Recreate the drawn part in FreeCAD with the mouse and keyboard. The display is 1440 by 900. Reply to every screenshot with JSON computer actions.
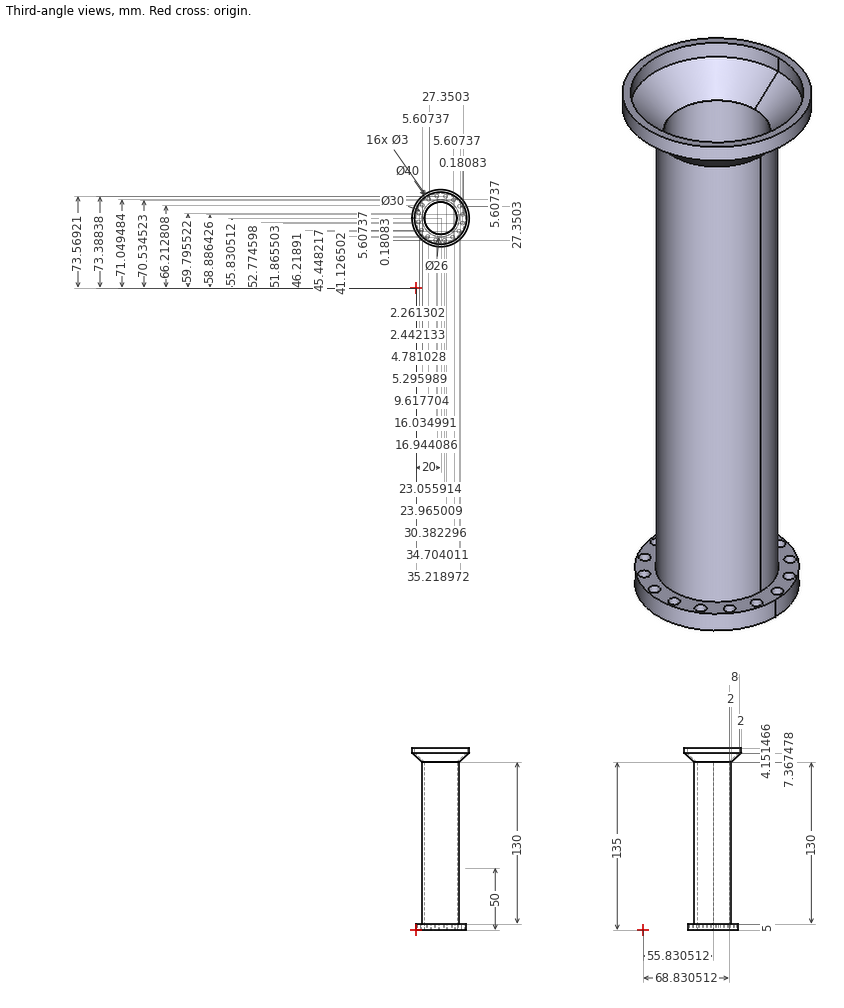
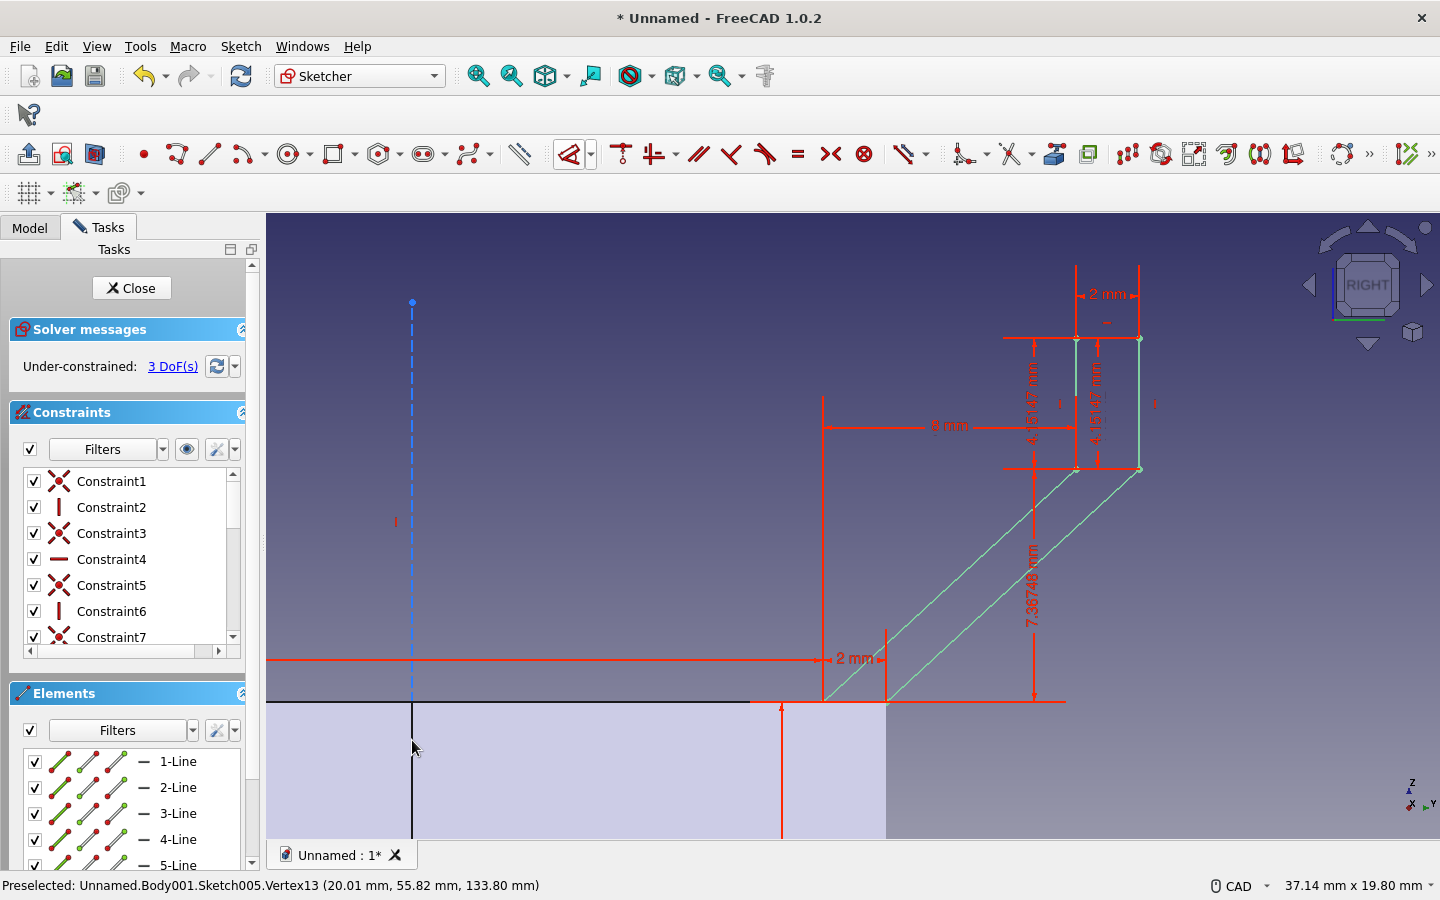
{"action": "key", "text": "l"}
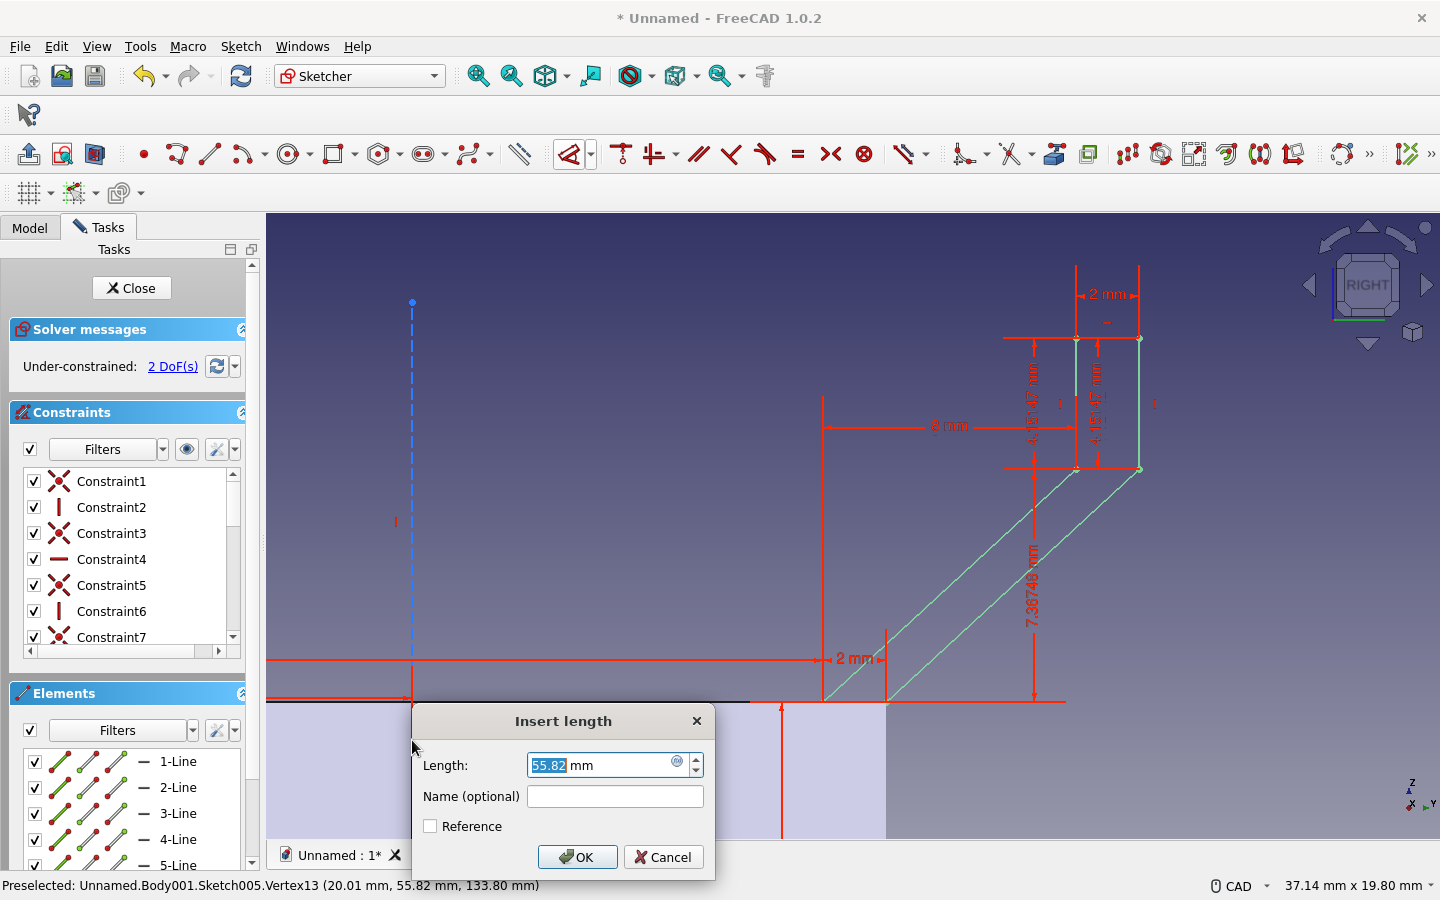
{"action": "type", "text": "55.830512"}
{"action": "key", "text": "Return"}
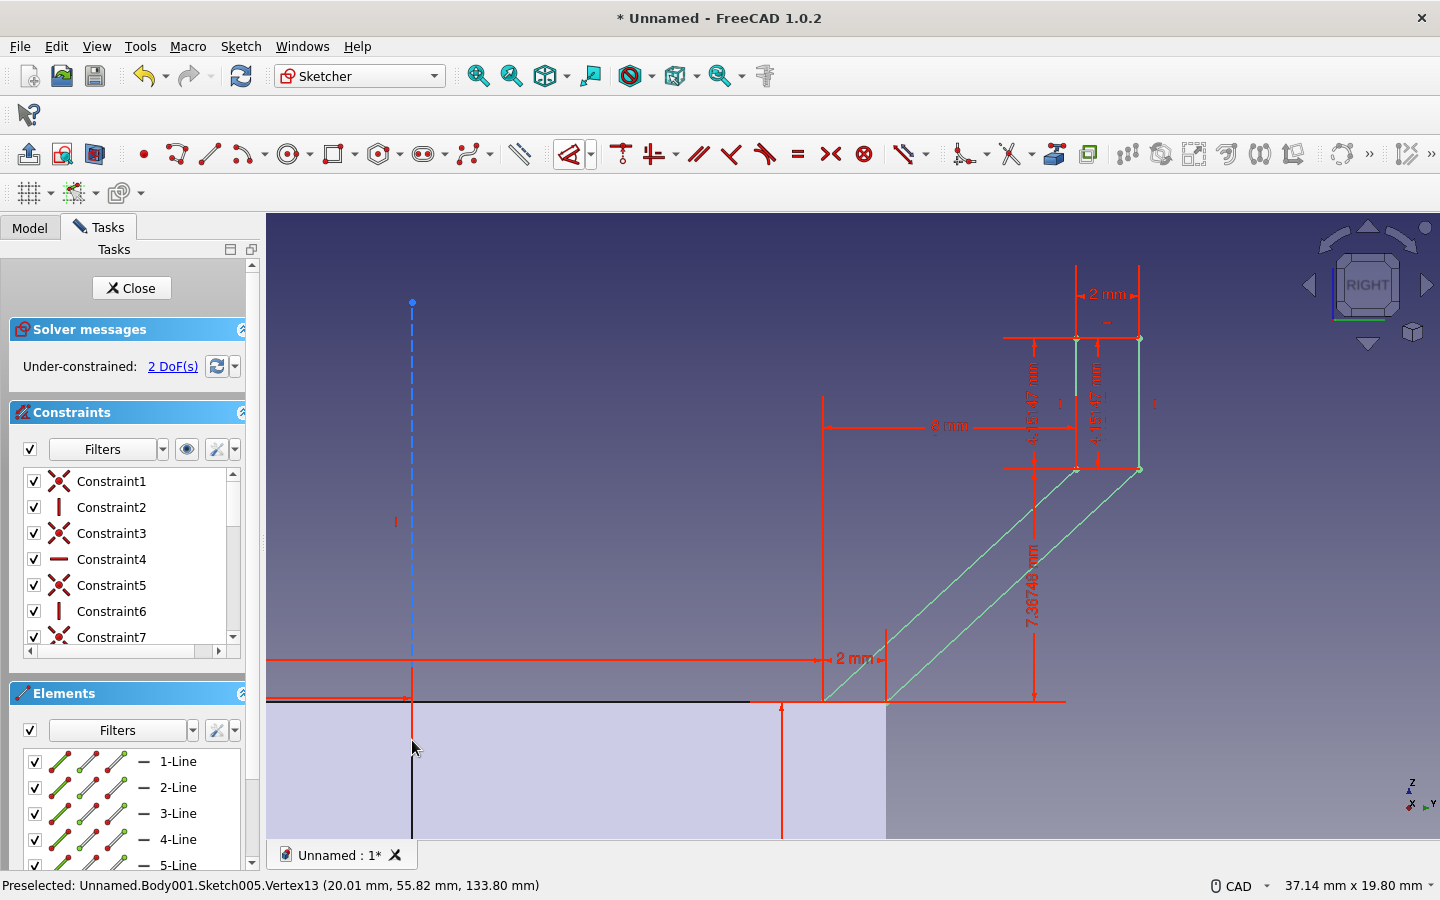
{"action": "left_click", "coordinate": [132, 288]}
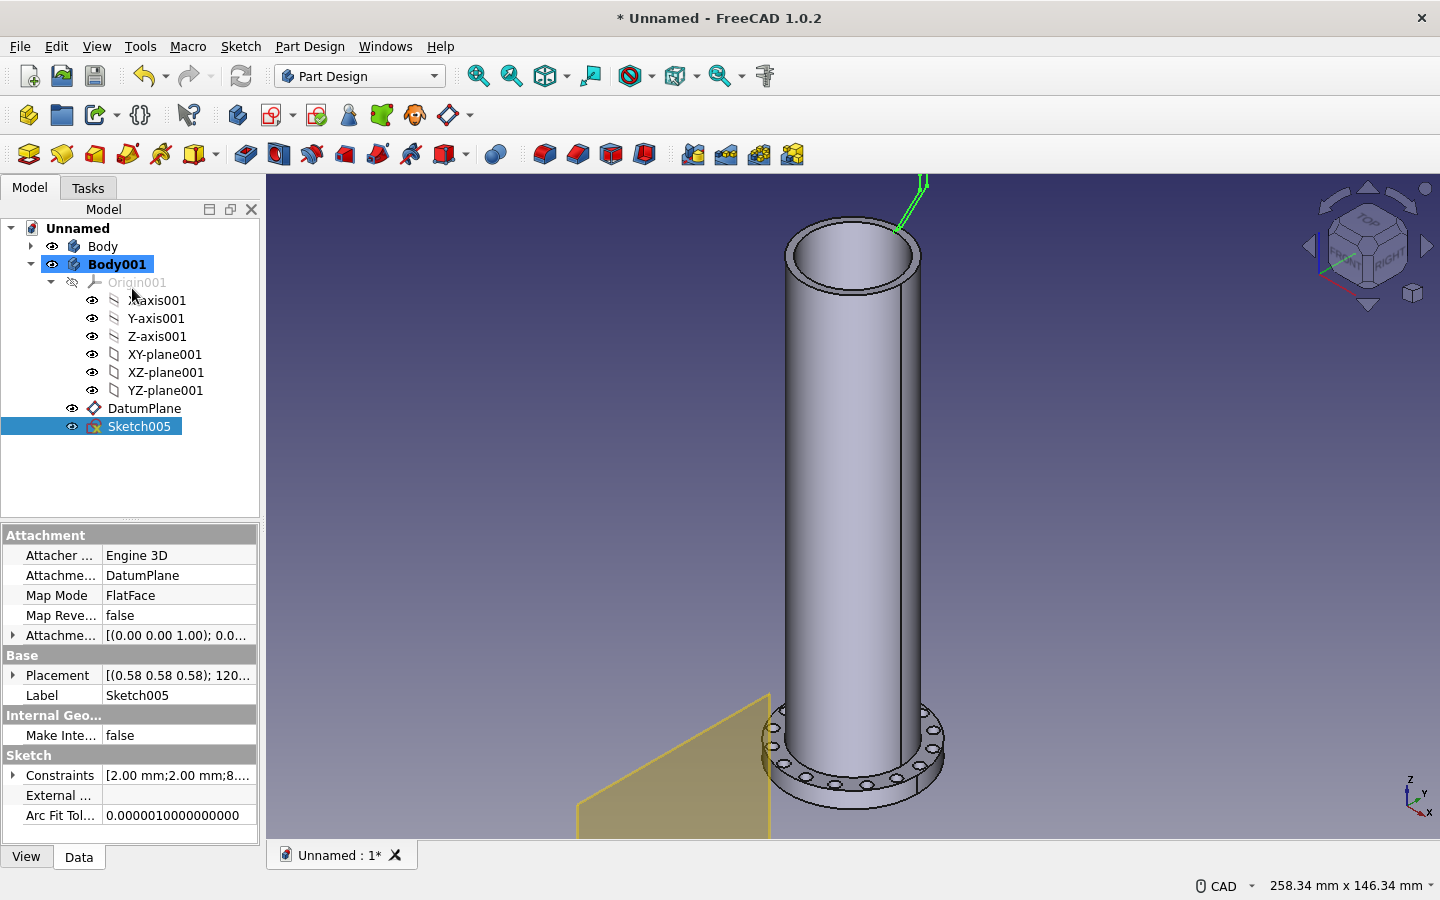
{"action": "left_click", "coordinate": [62, 154]}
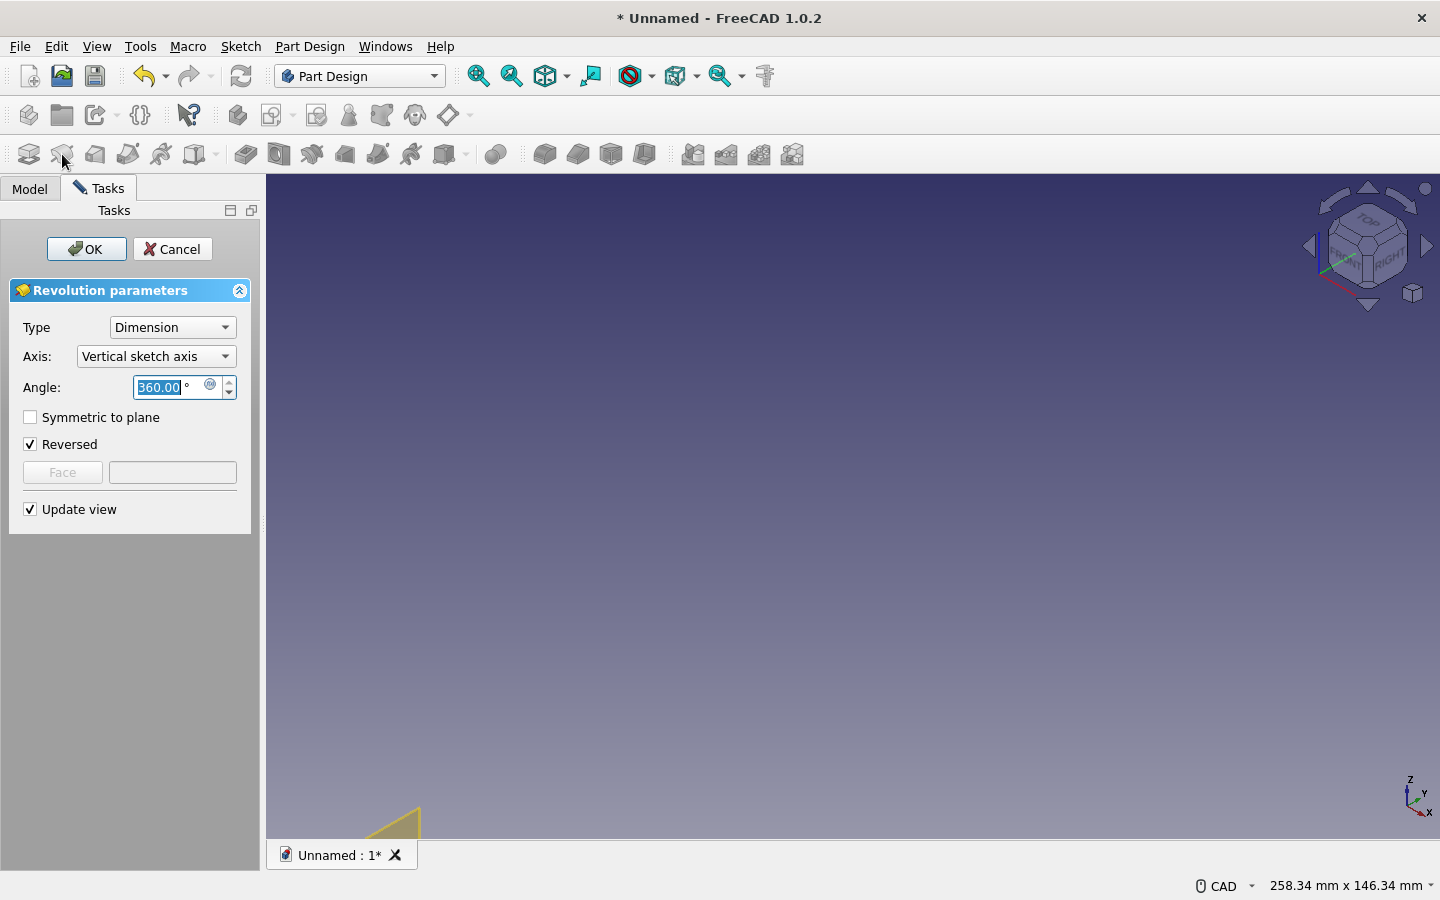
{"action": "left_click", "coordinate": [157, 356]}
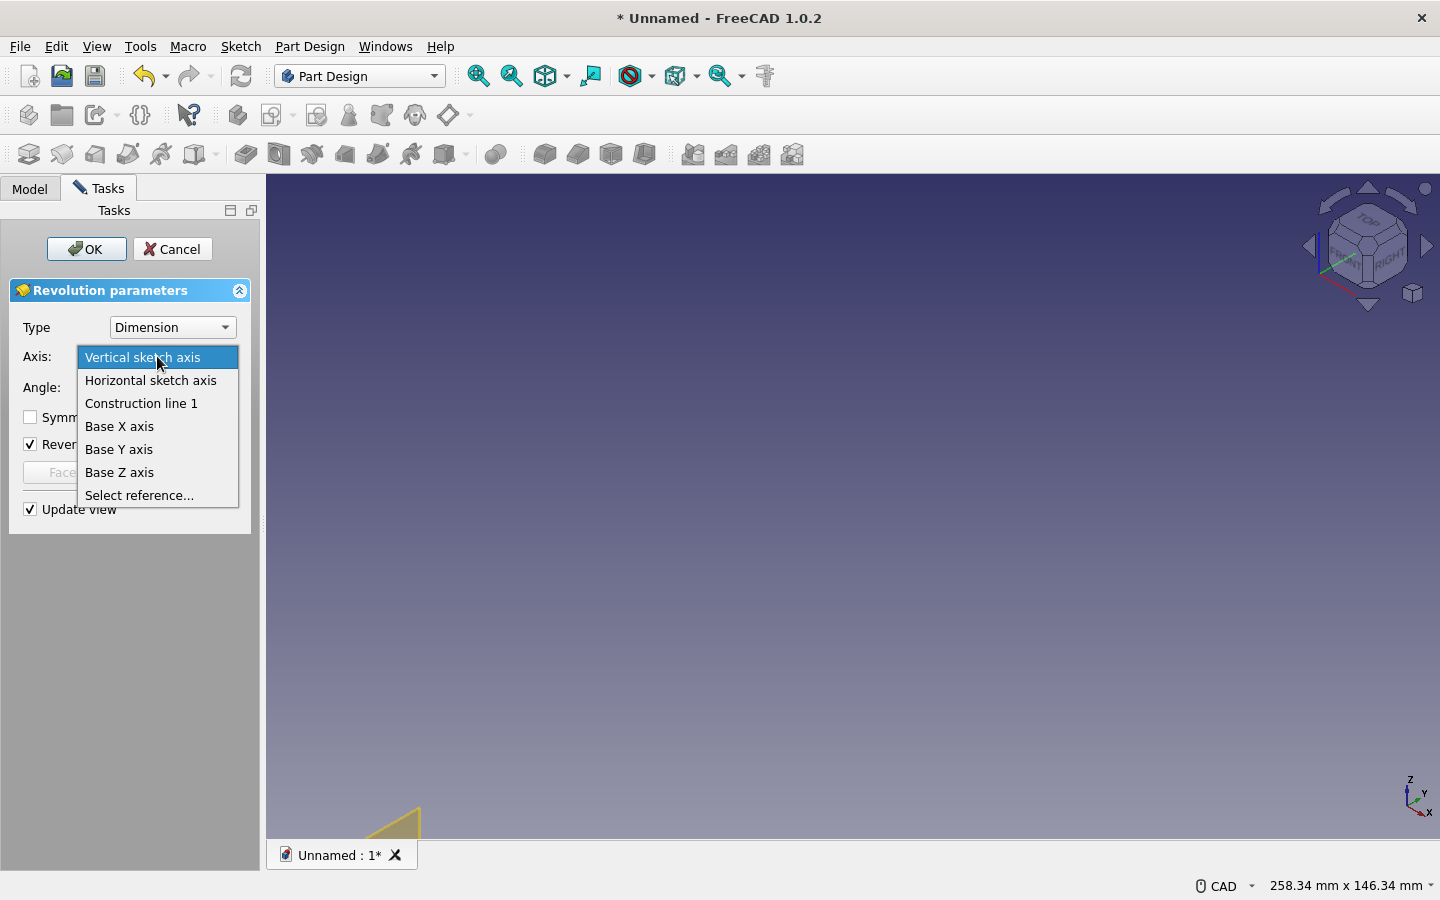
{"action": "left_click", "coordinate": [156, 404]}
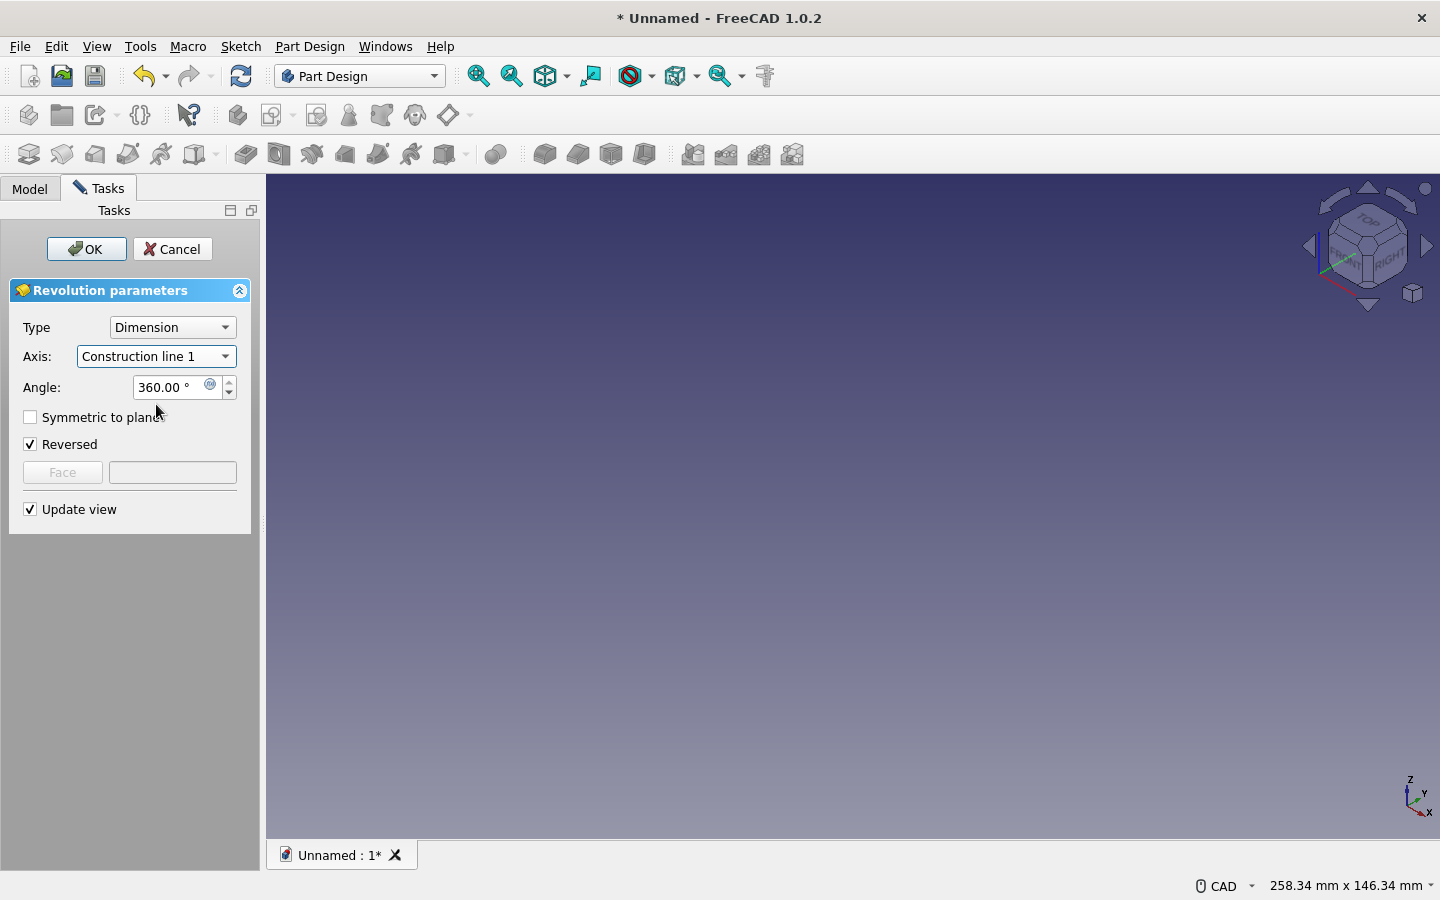
{"action": "left_click", "coordinate": [87, 249]}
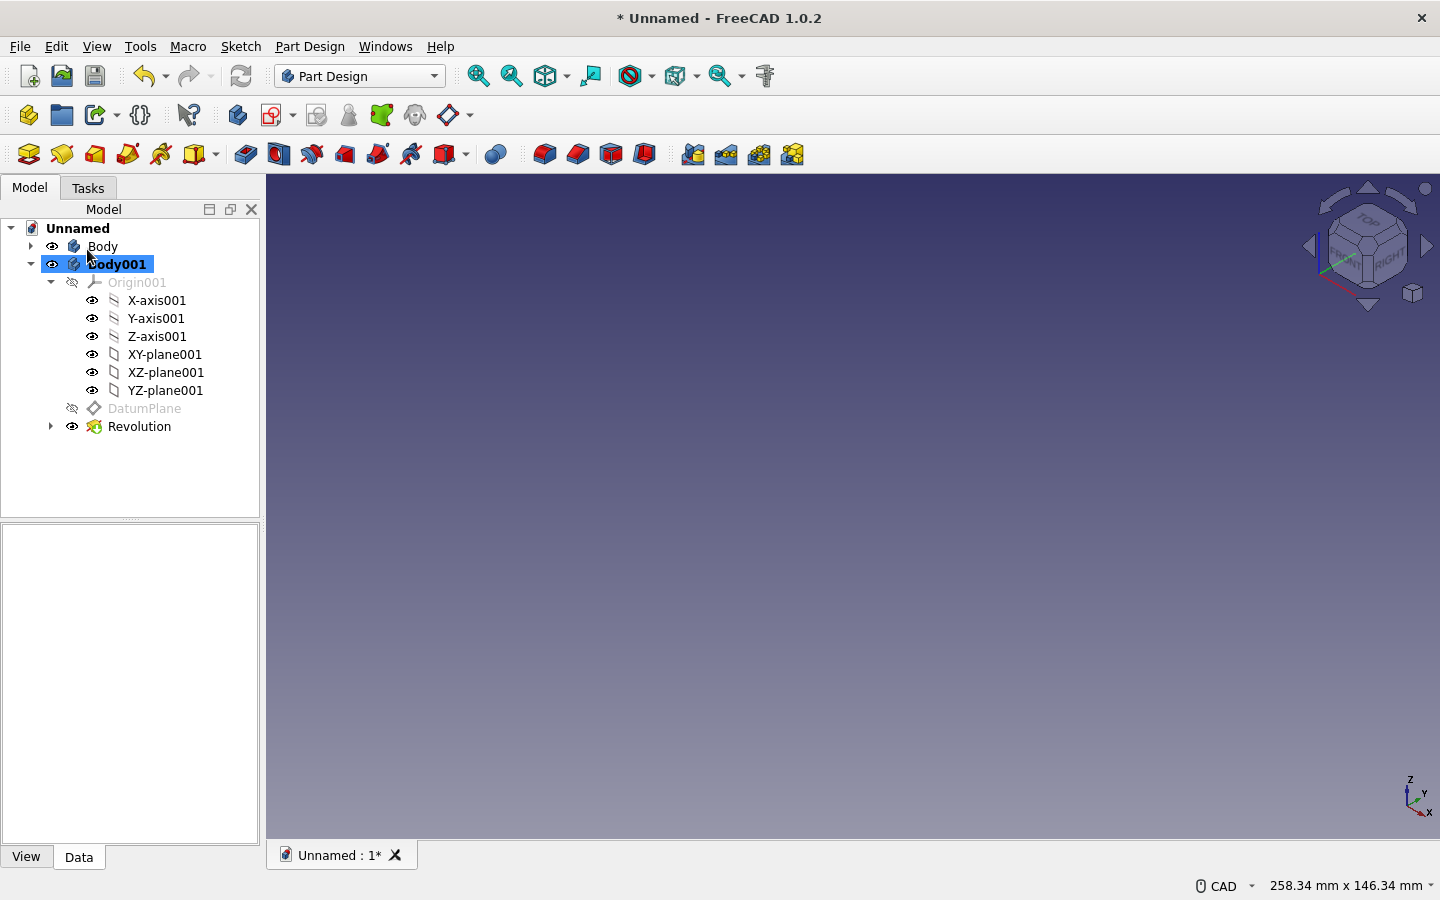
{"action": "left_click", "coordinate": [479, 76]}